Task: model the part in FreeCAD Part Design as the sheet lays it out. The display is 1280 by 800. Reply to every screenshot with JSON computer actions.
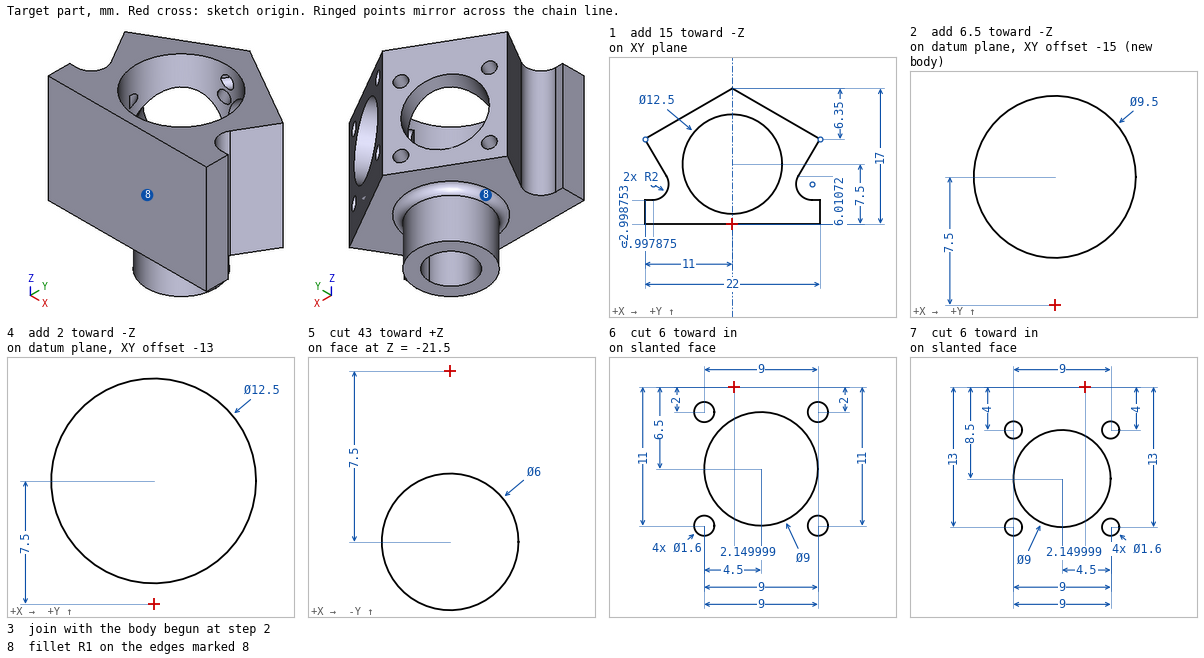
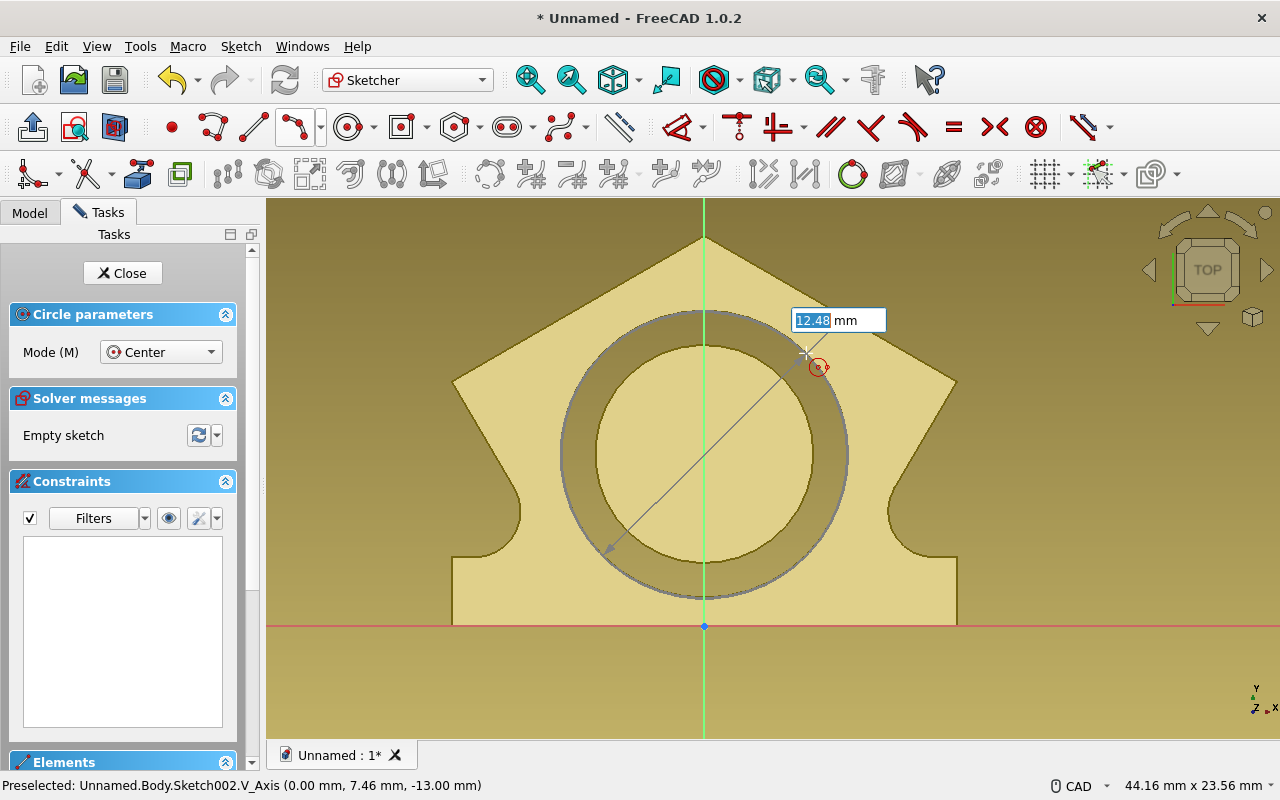
{"action": "type", "text": "12.5"}
{"action": "key", "text": "Return"}
{"action": "key", "text": "Escape"}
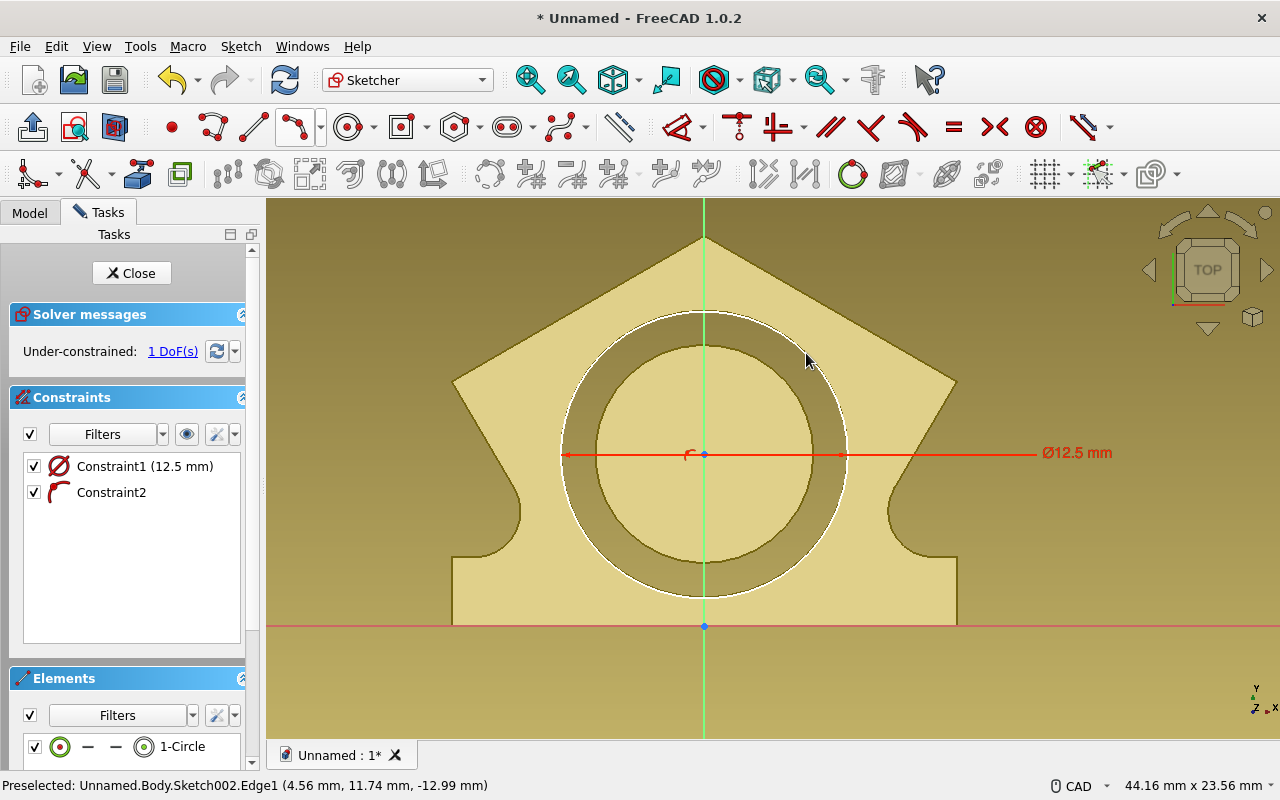
{"action": "left_click", "coordinate": [676, 128]}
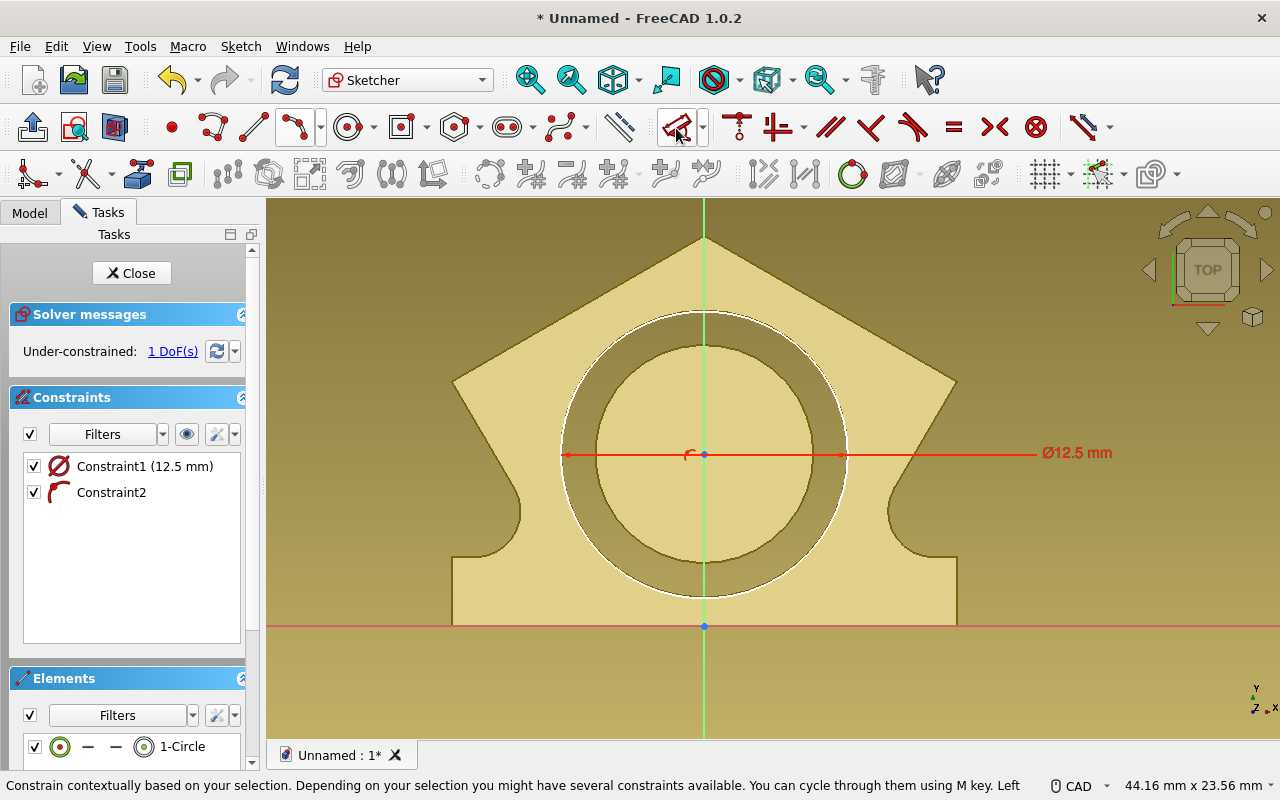
{"action": "left_click", "coordinate": [704, 455]}
{"action": "left_click", "coordinate": [738, 541]}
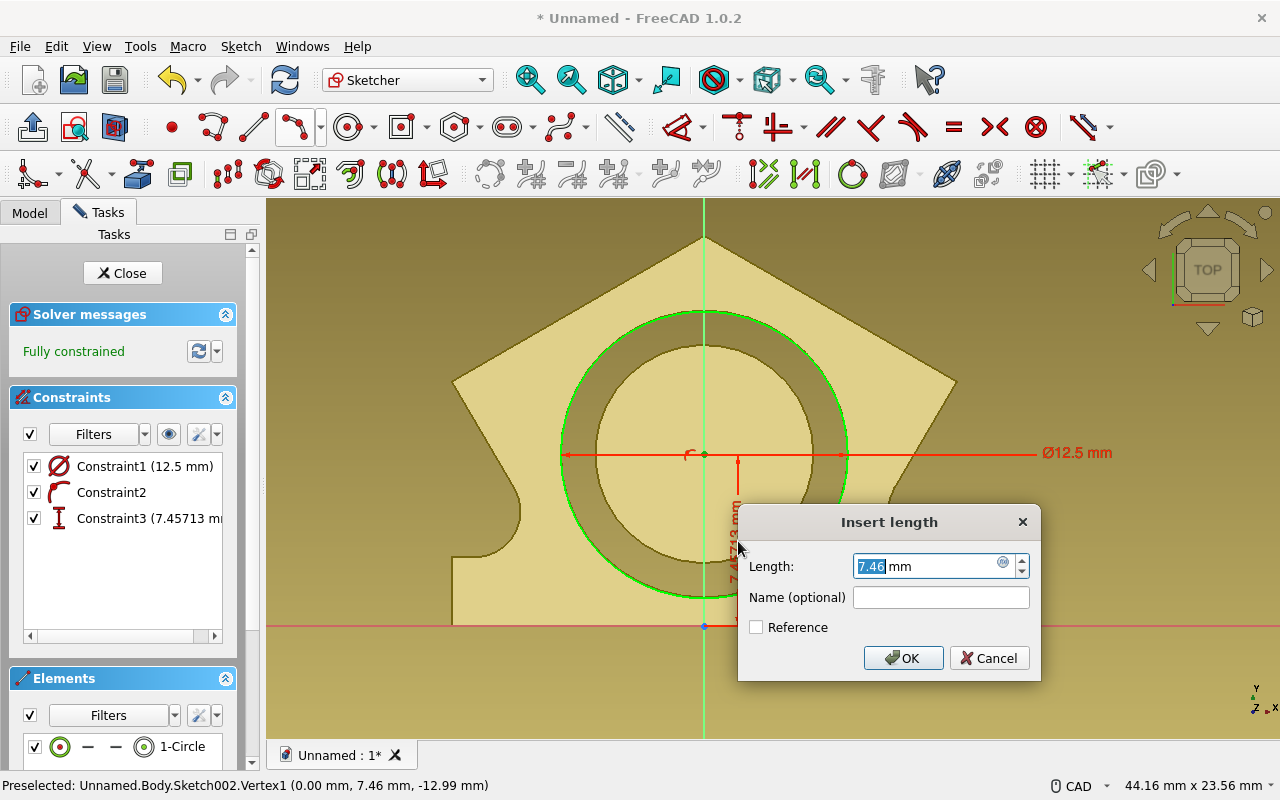
{"action": "type", "text": "7.5"}
{"action": "key", "text": "Return"}
{"action": "key", "text": "Escape"}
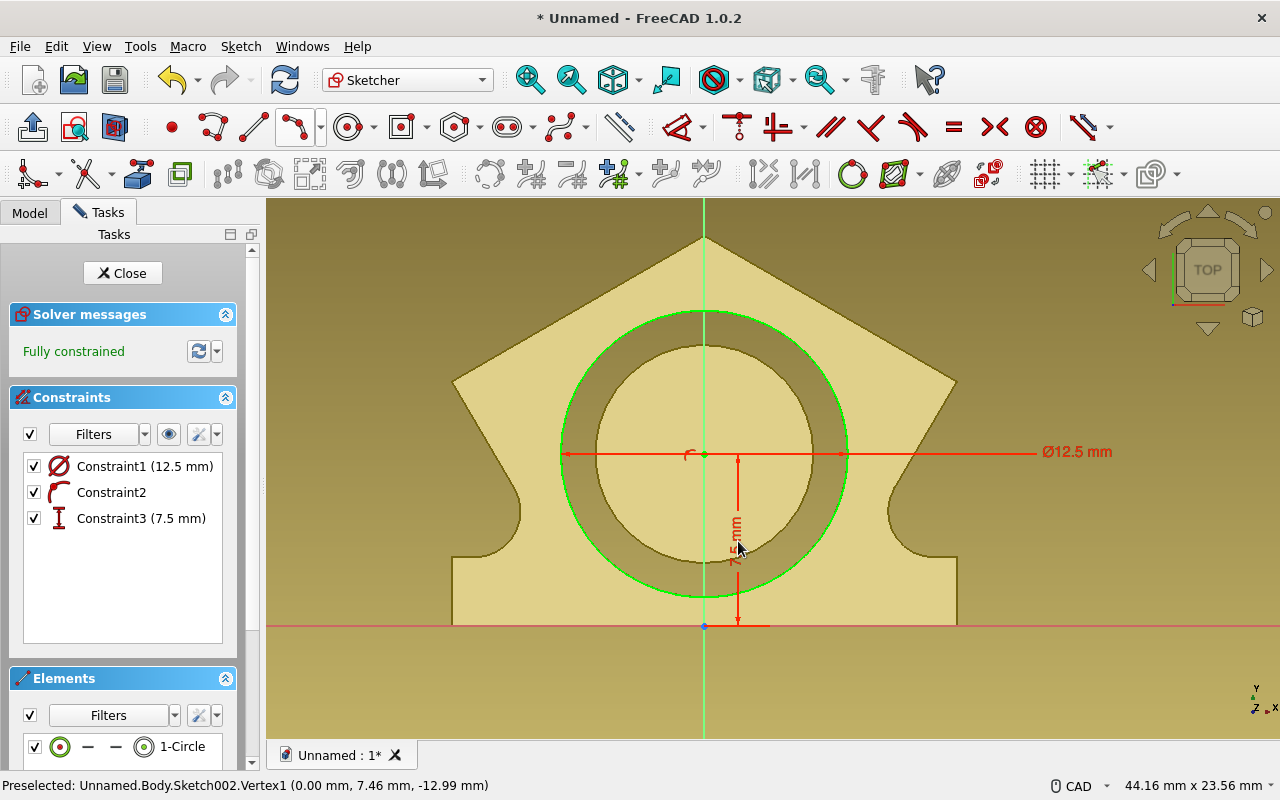
{"action": "left_click", "coordinate": [123, 273]}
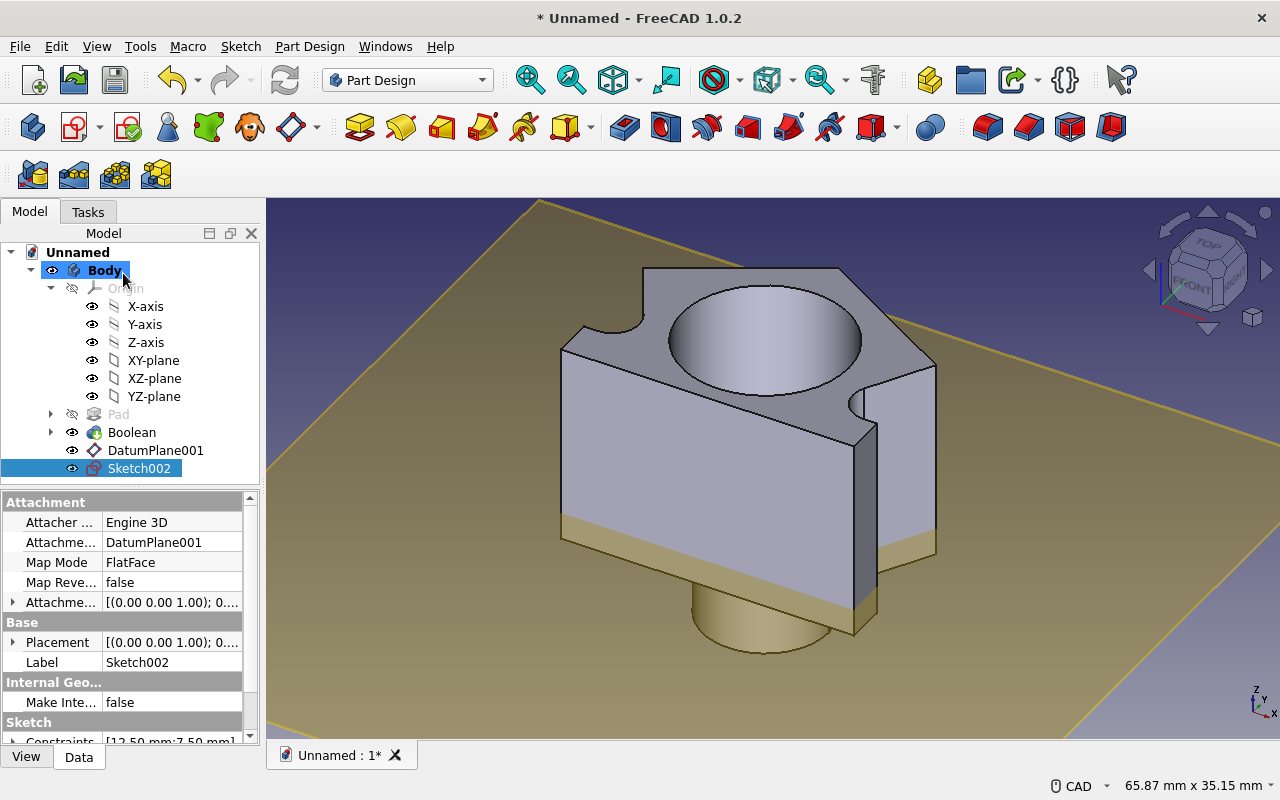
{"action": "left_click", "coordinate": [360, 128]}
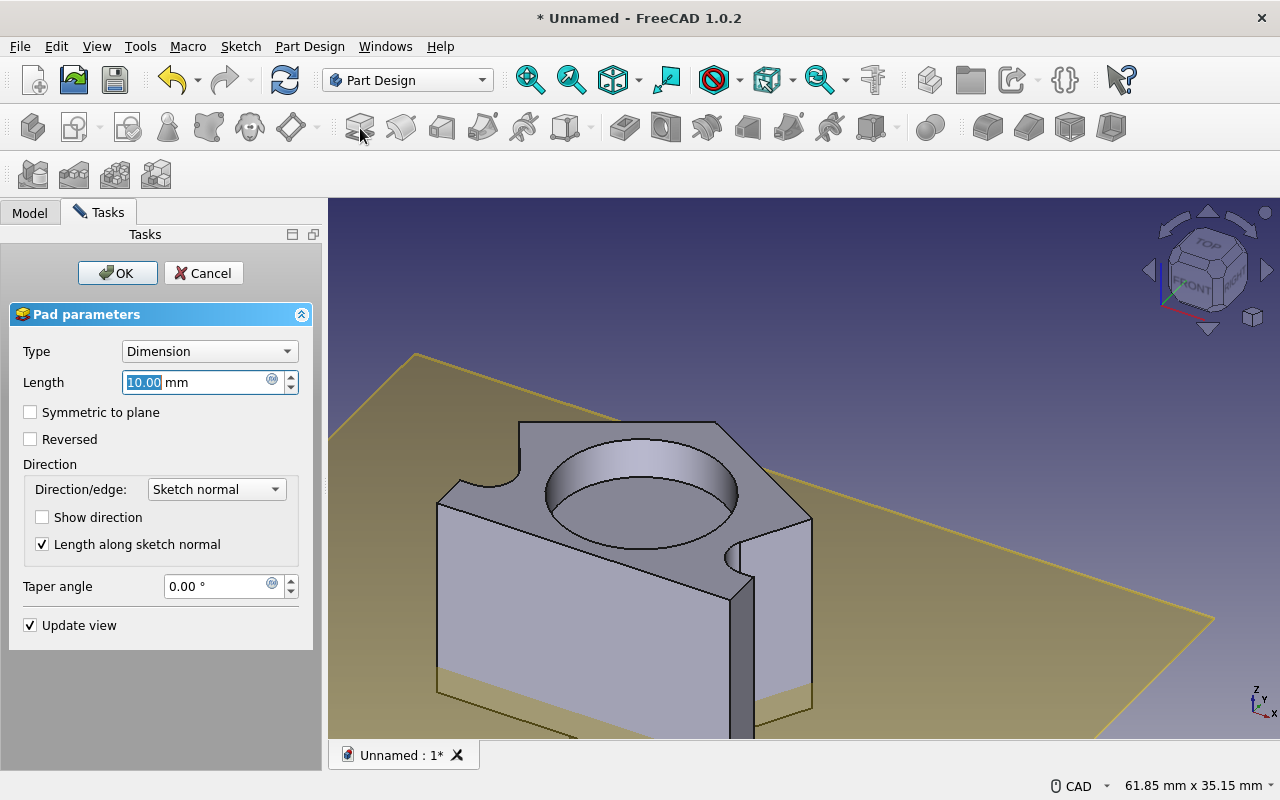
{"action": "type", "text": "2"}
{"action": "key", "text": "Tab"}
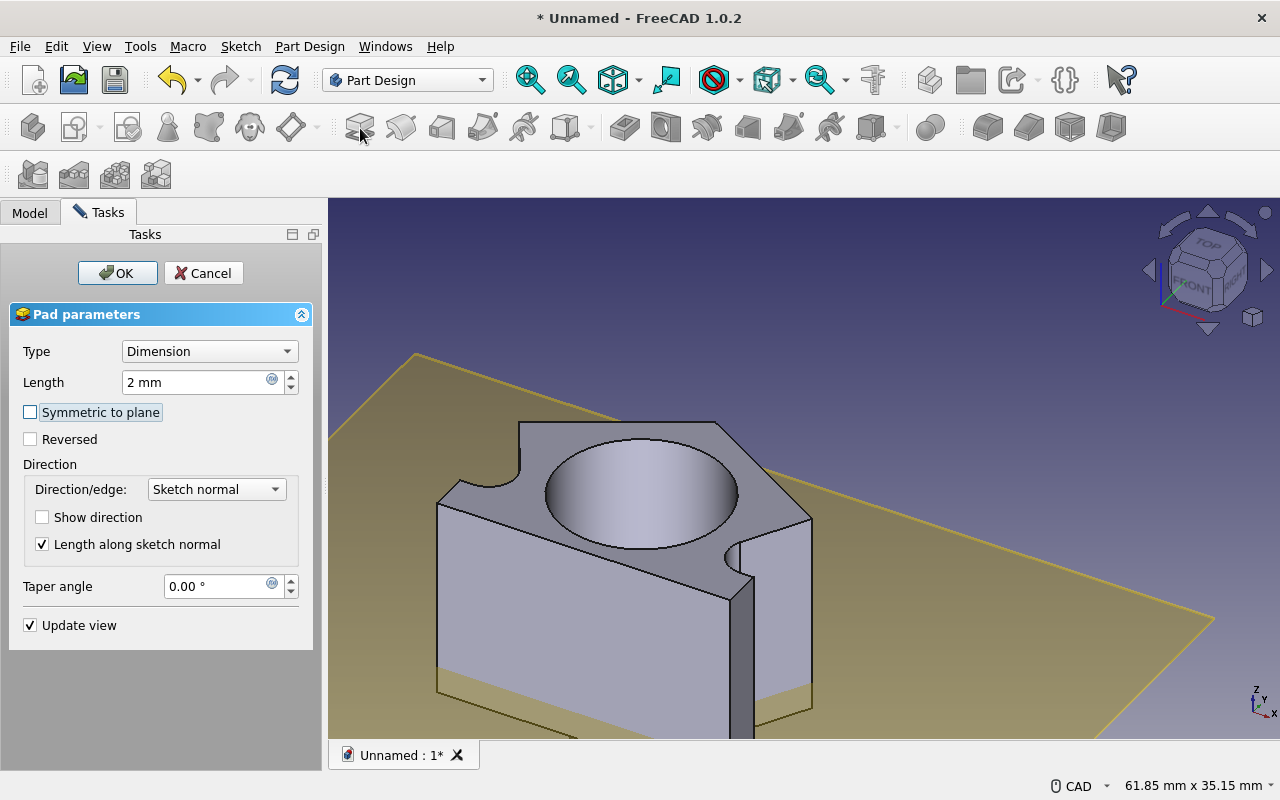
{"action": "left_click", "coordinate": [31, 439]}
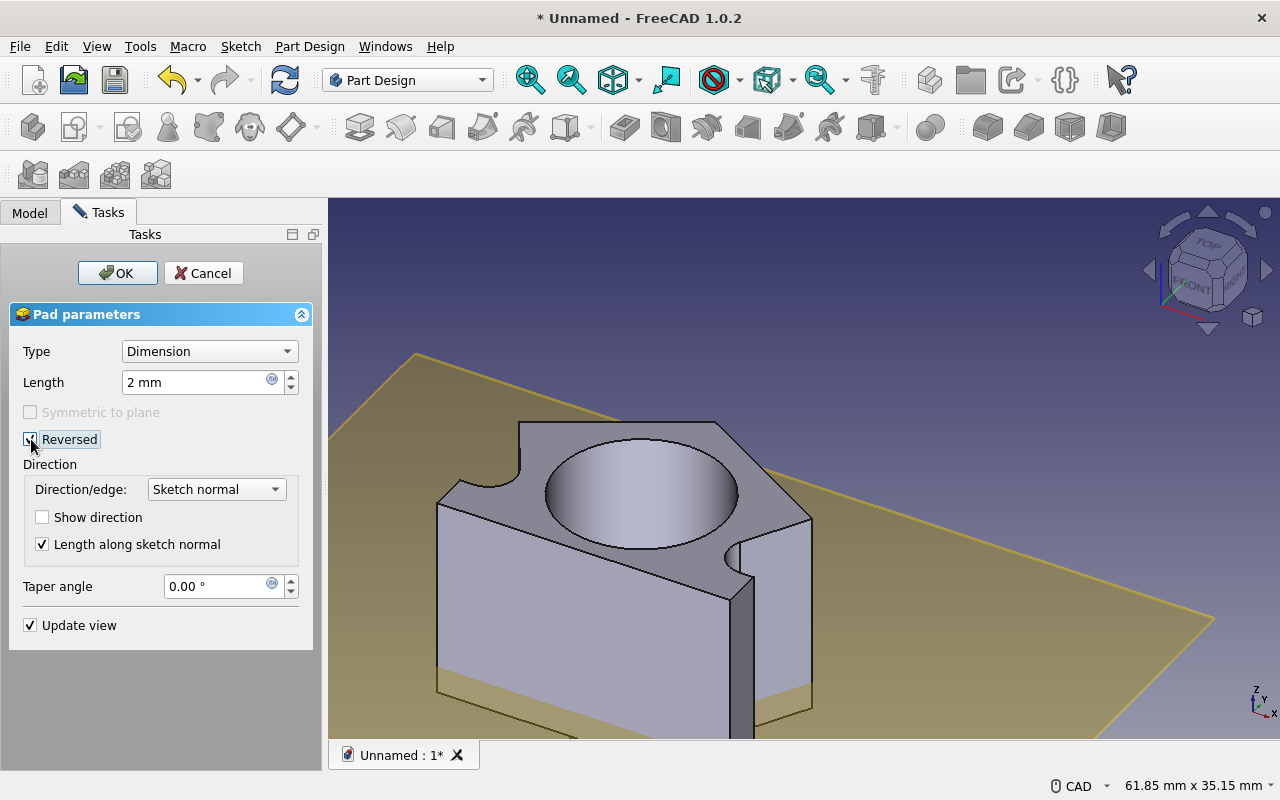
{"action": "left_click", "coordinate": [118, 273]}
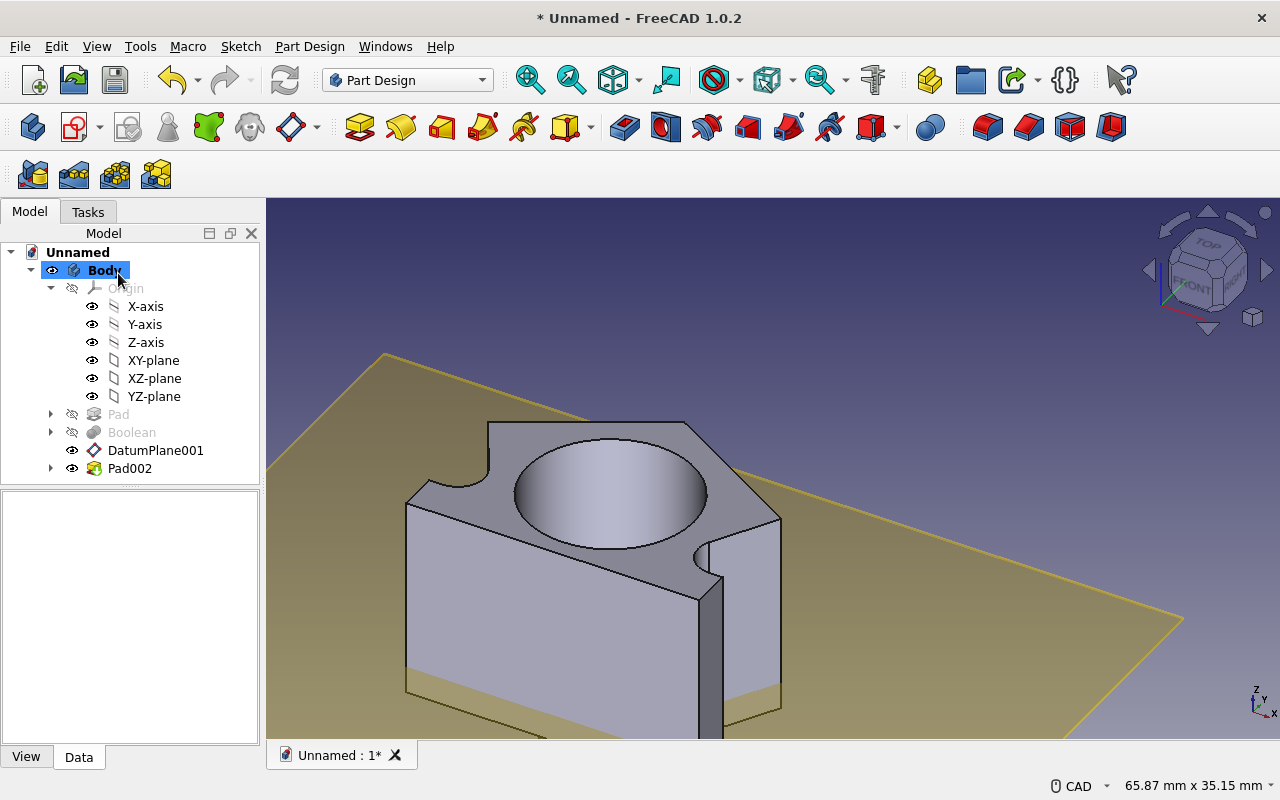
{"action": "left_click", "coordinate": [117, 450]}
{"action": "key", "text": "space"}